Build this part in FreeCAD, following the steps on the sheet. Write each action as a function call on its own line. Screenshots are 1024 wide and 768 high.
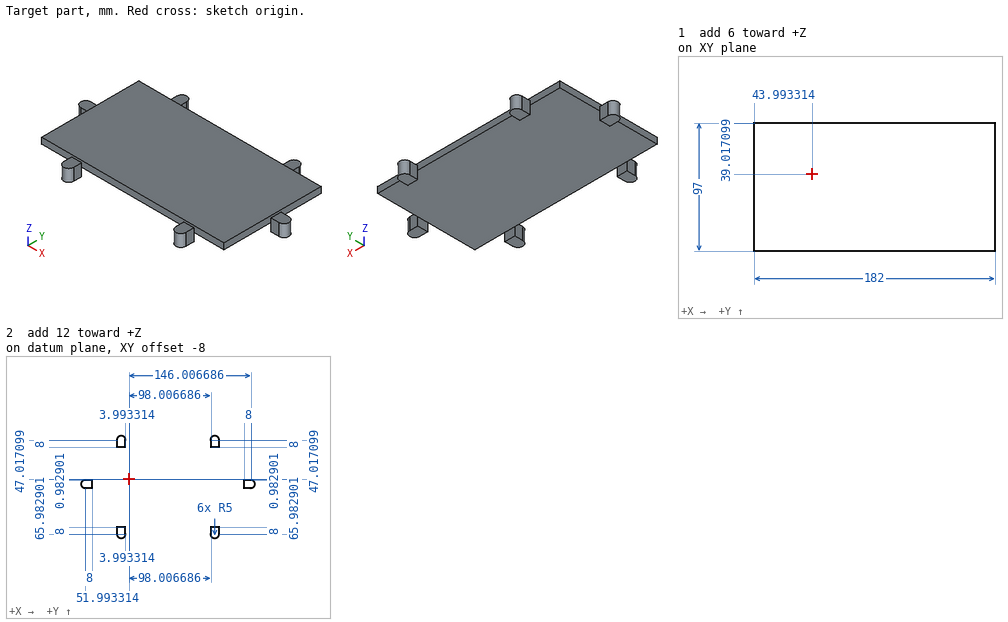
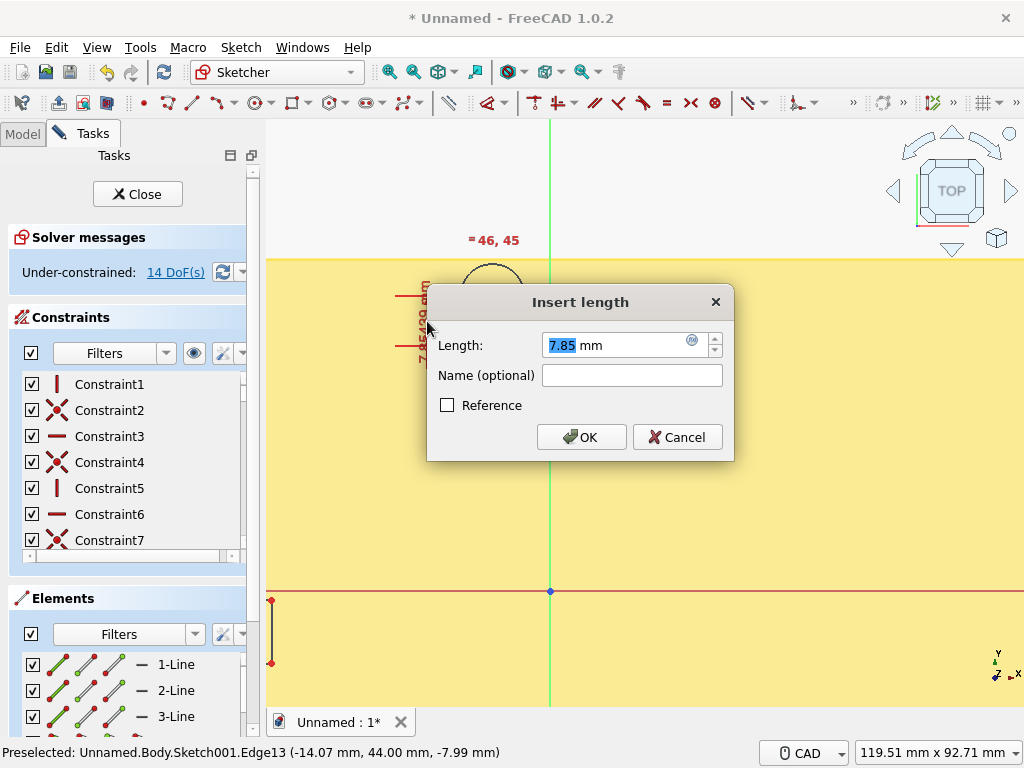
text(8)
key(Return)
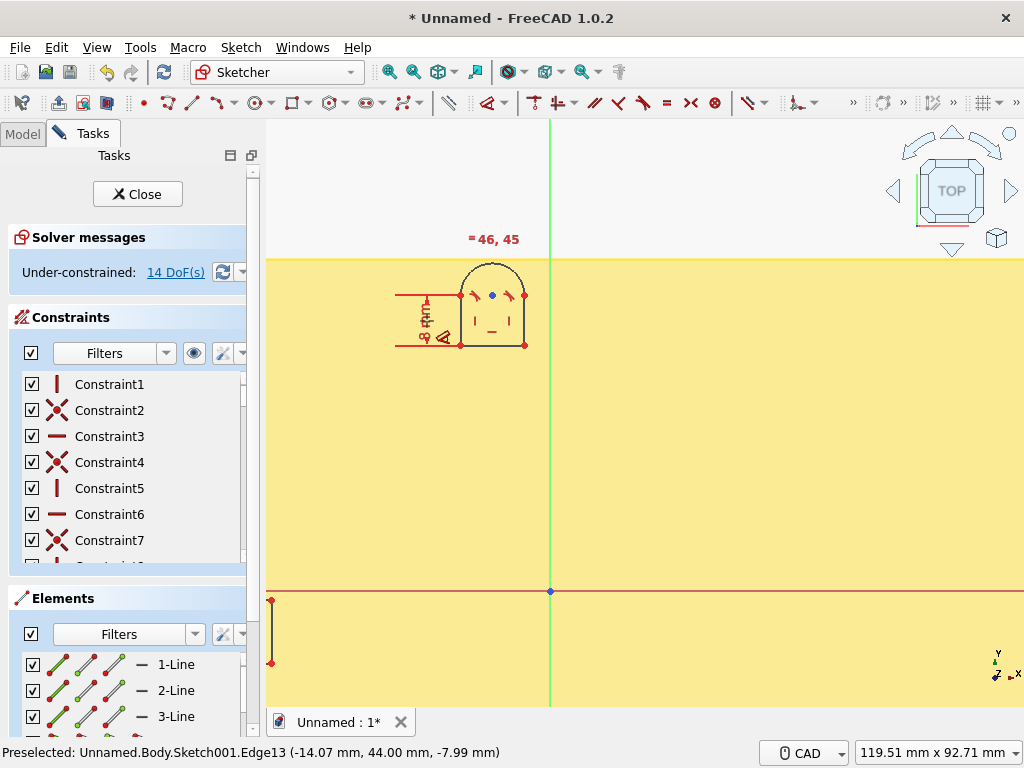
scroll(459, 310, down, 6)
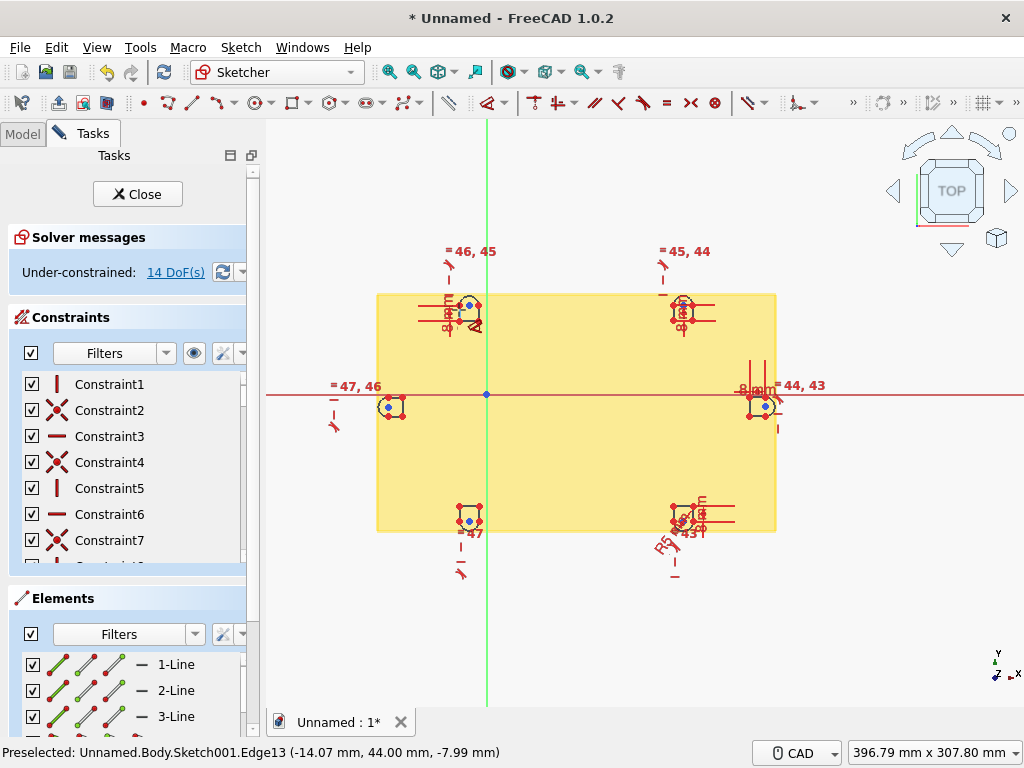
scroll(392, 417, up, 6)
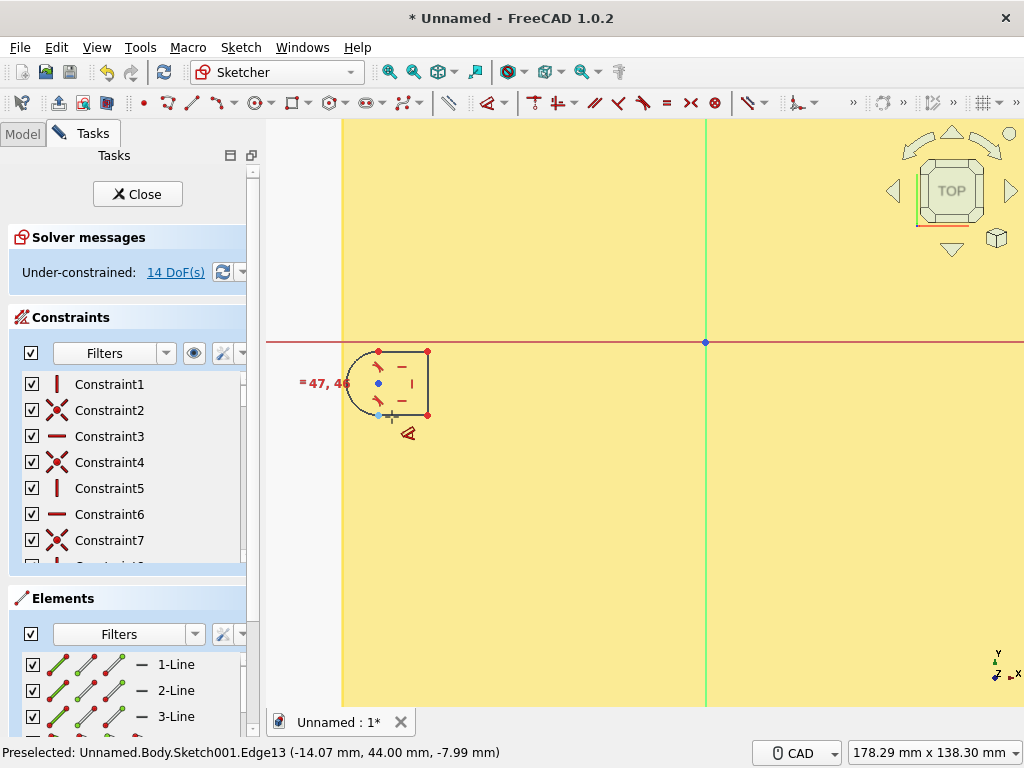
click(393, 415)
click(403, 449)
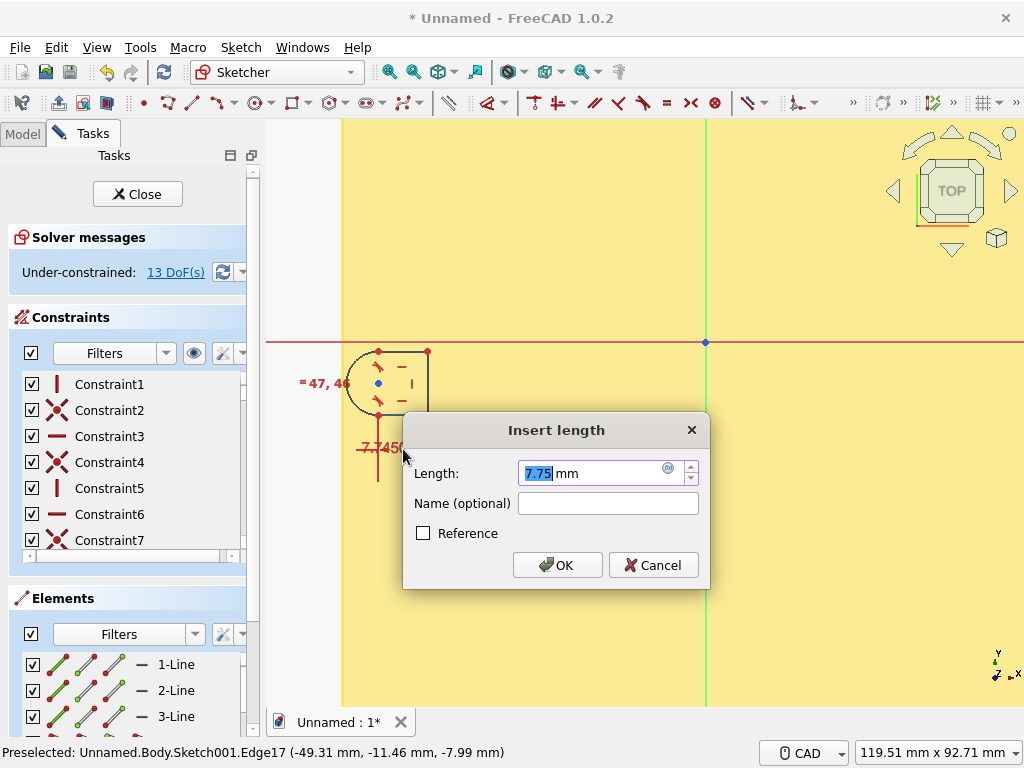
text(8)
key(Return)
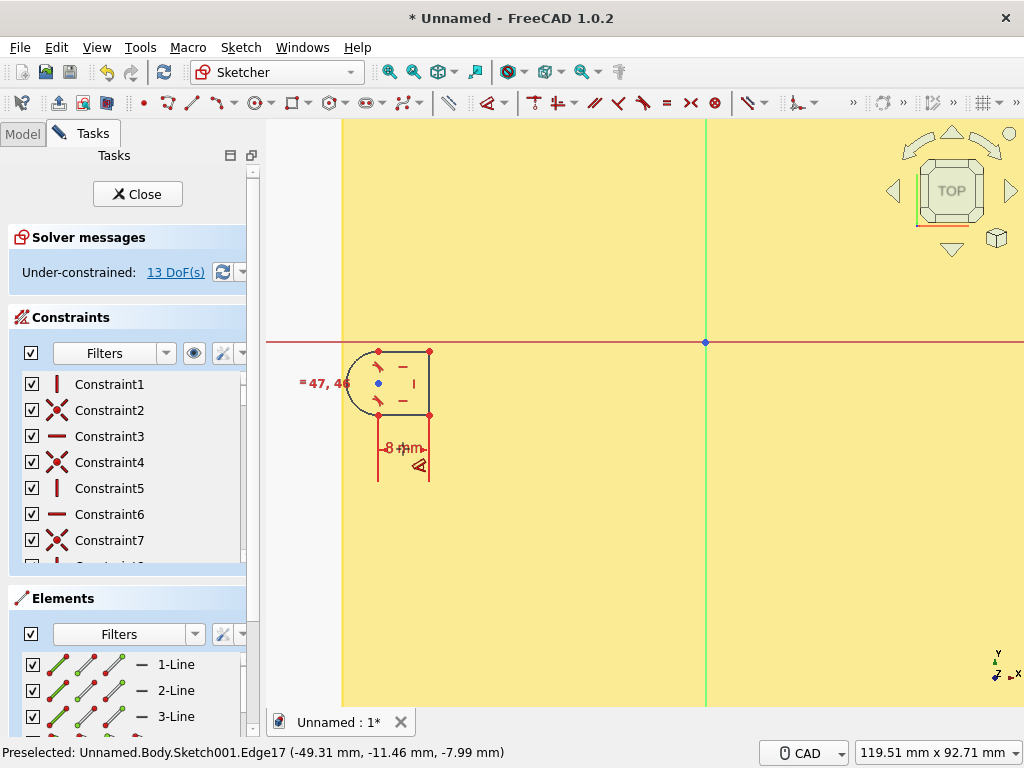
scroll(392, 418, down, 6)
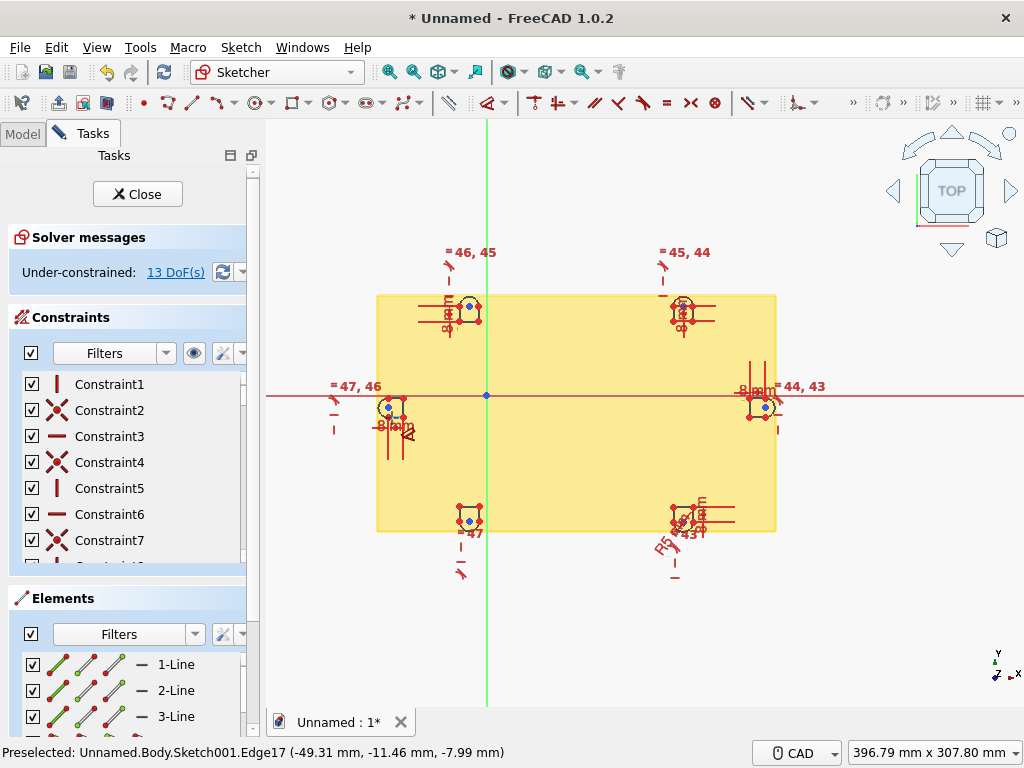
scroll(479, 517, up, 6)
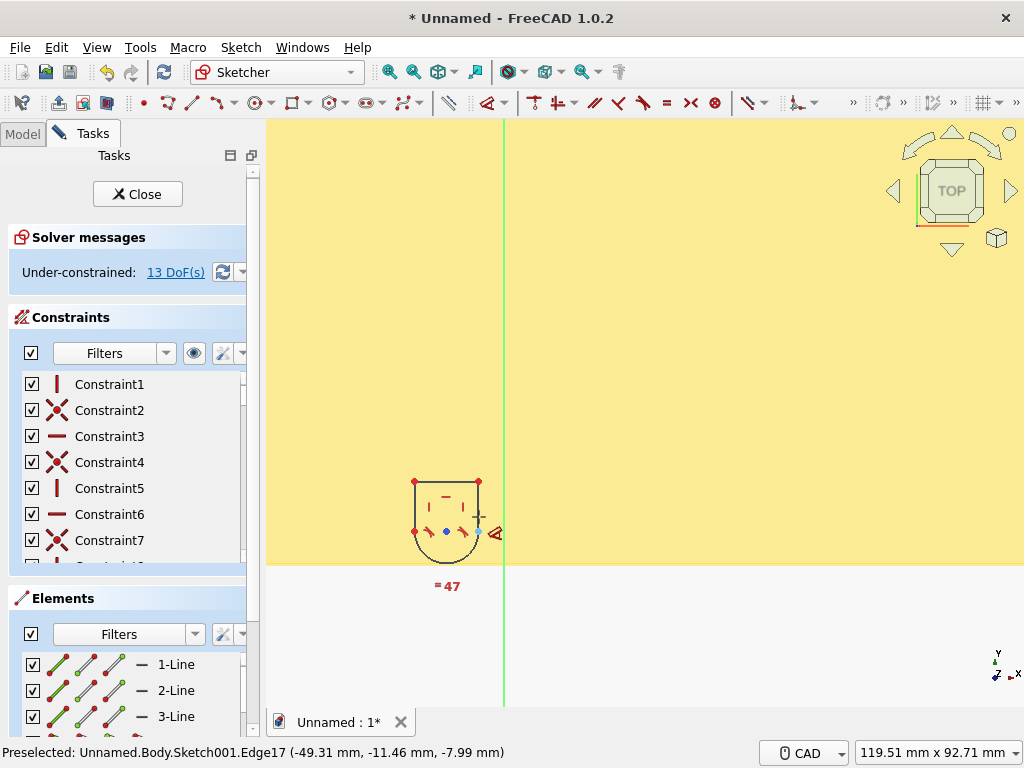
click(478, 517)
click(444, 507)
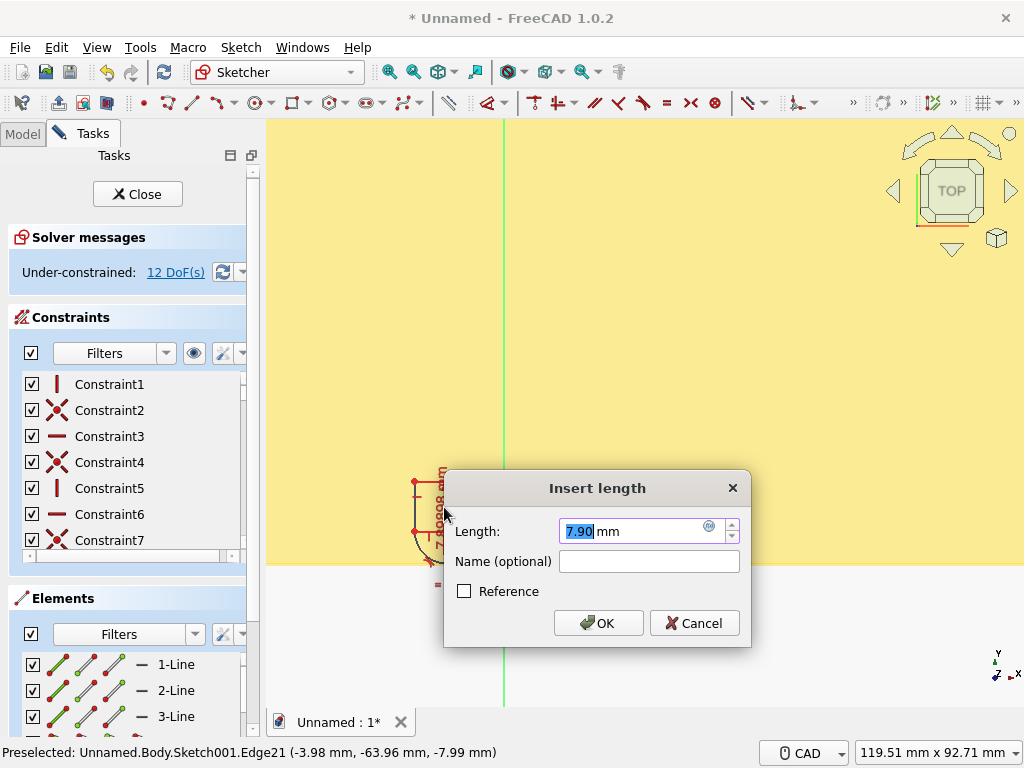
text(8)
key(Return)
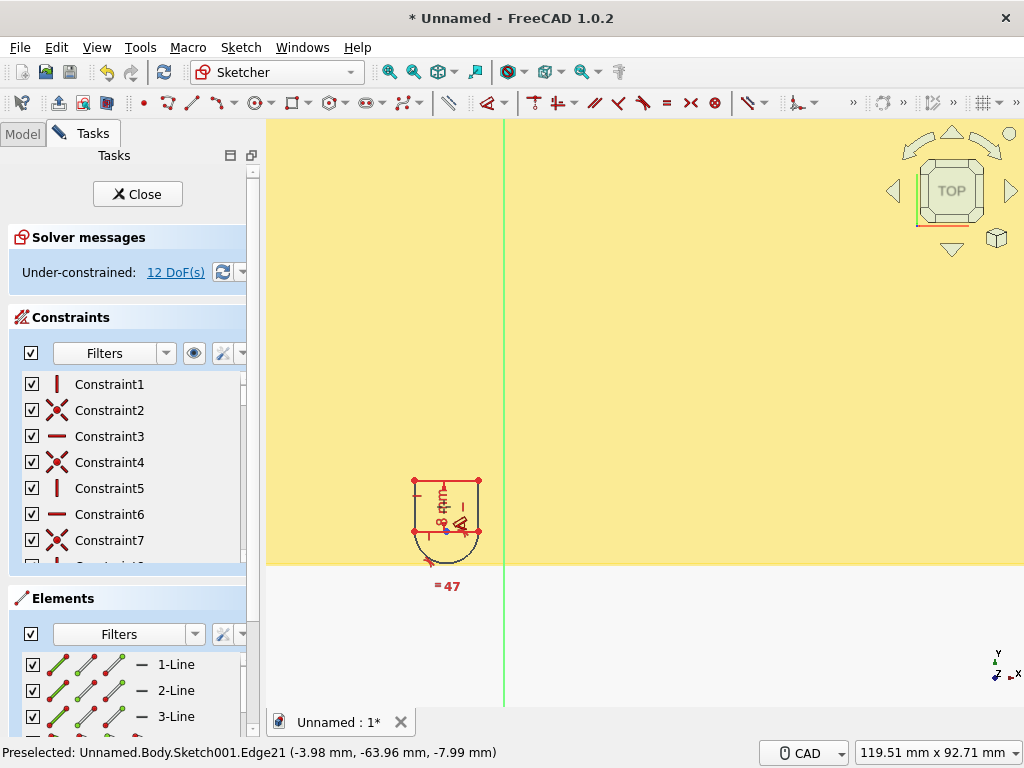
scroll(479, 517, down, 6)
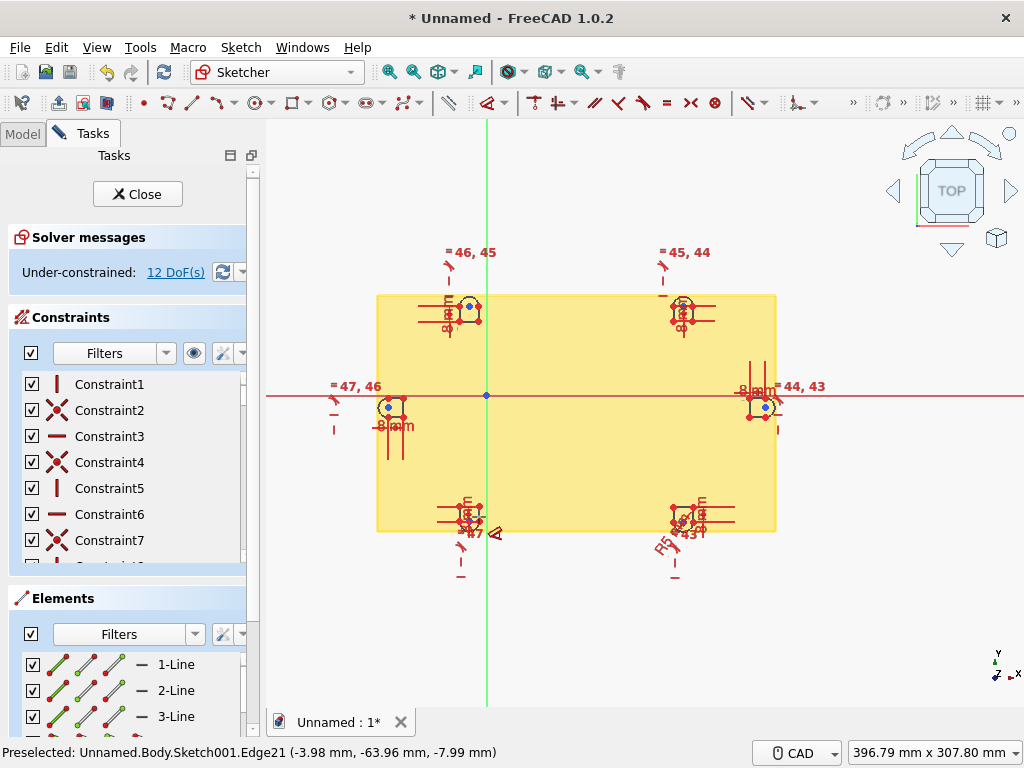
scroll(765, 398, up, 16)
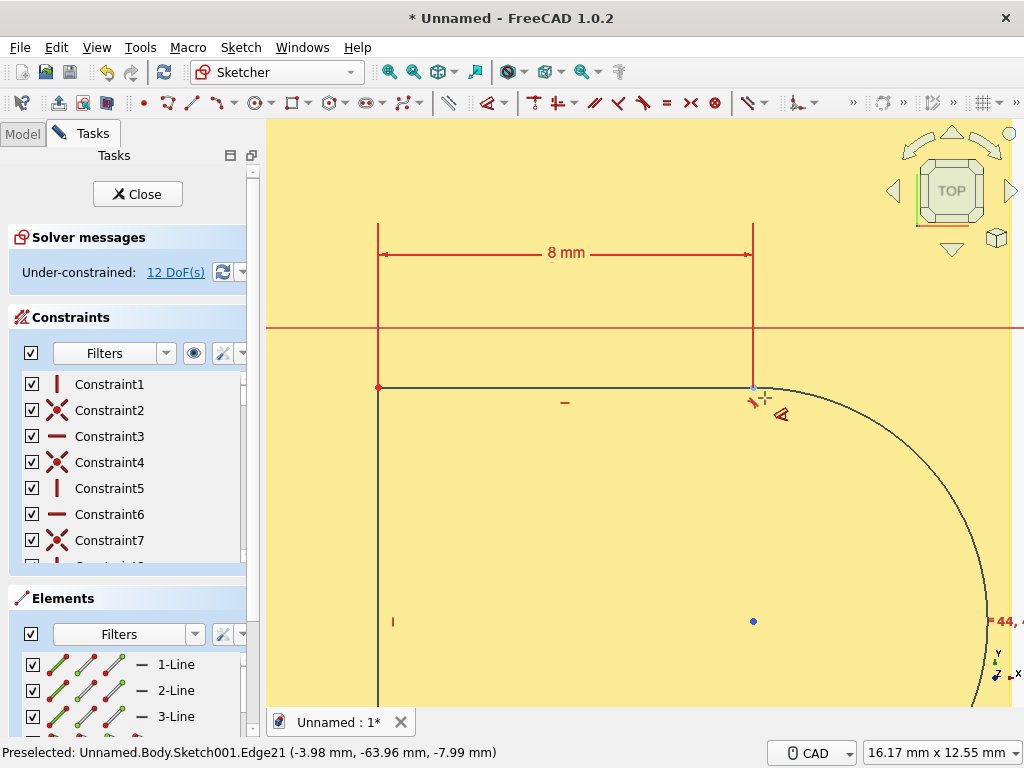
click(753, 388)
click(787, 358)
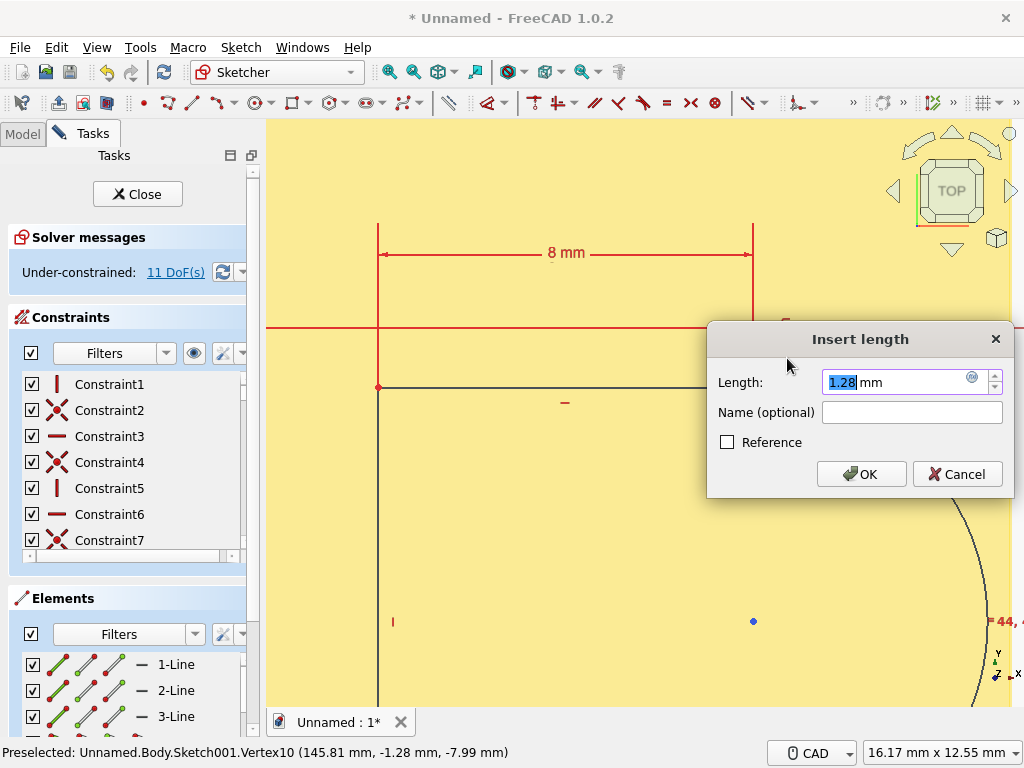
text(0.982901)
key(Return)